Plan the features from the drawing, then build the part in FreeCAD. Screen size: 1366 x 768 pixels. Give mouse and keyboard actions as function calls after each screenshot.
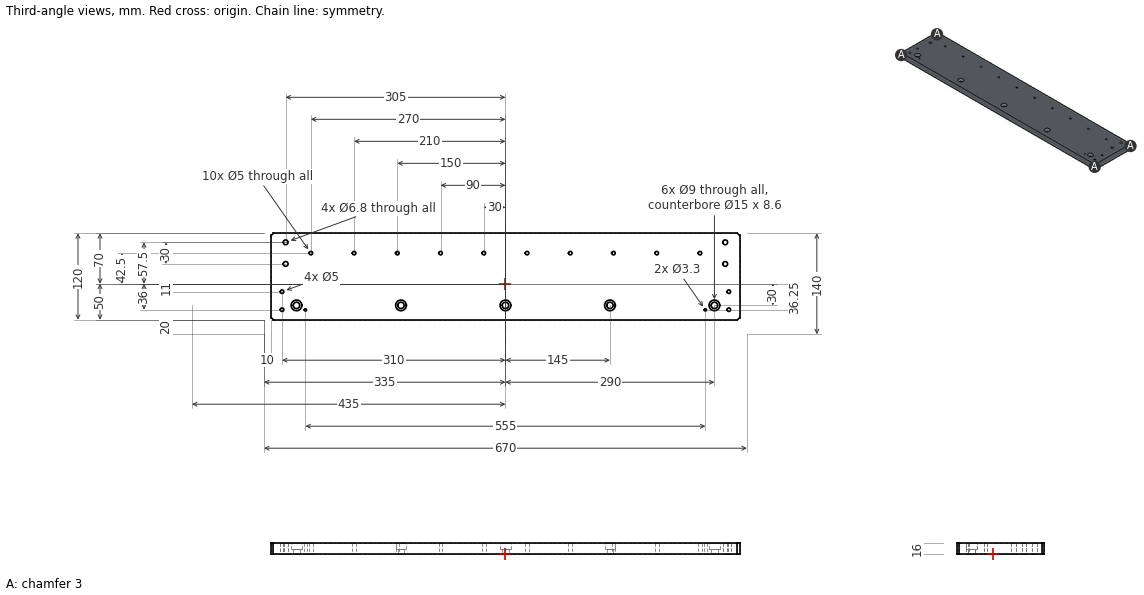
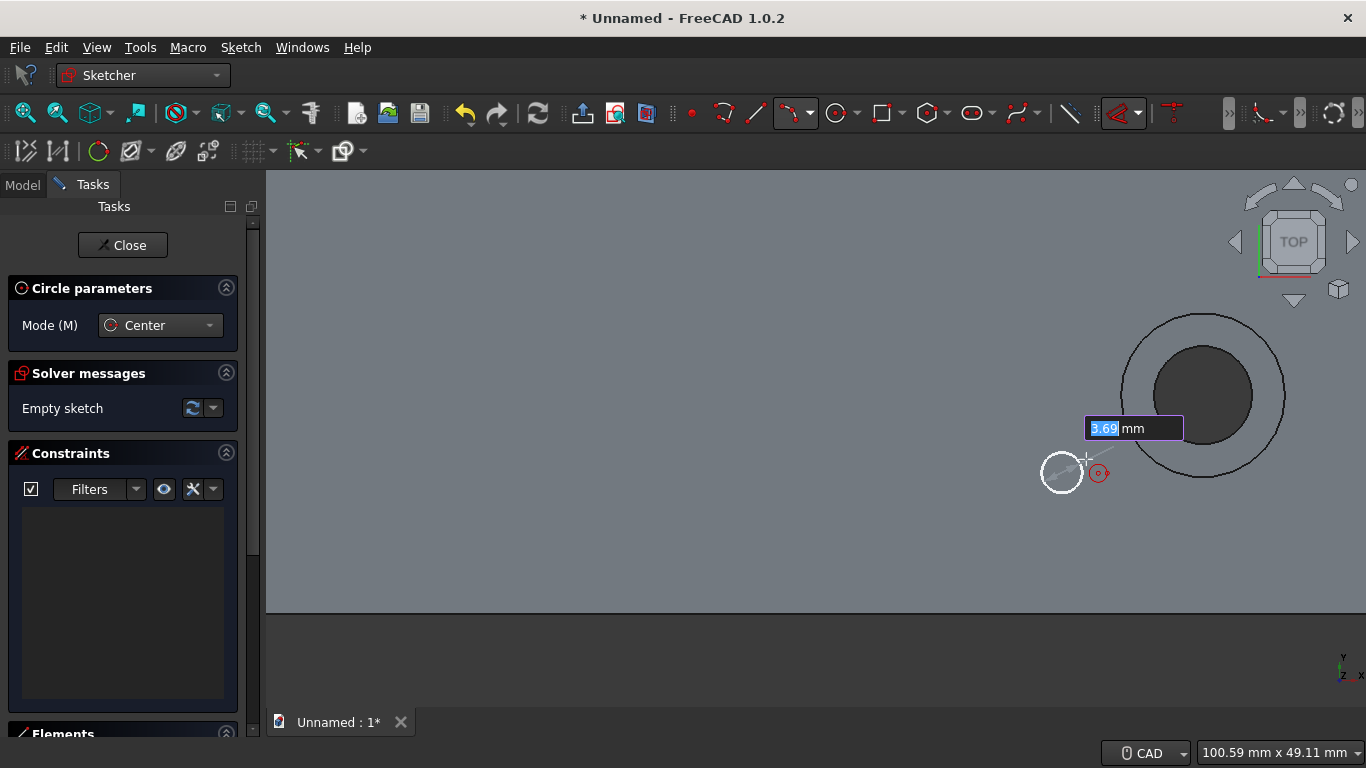
click(1079, 451)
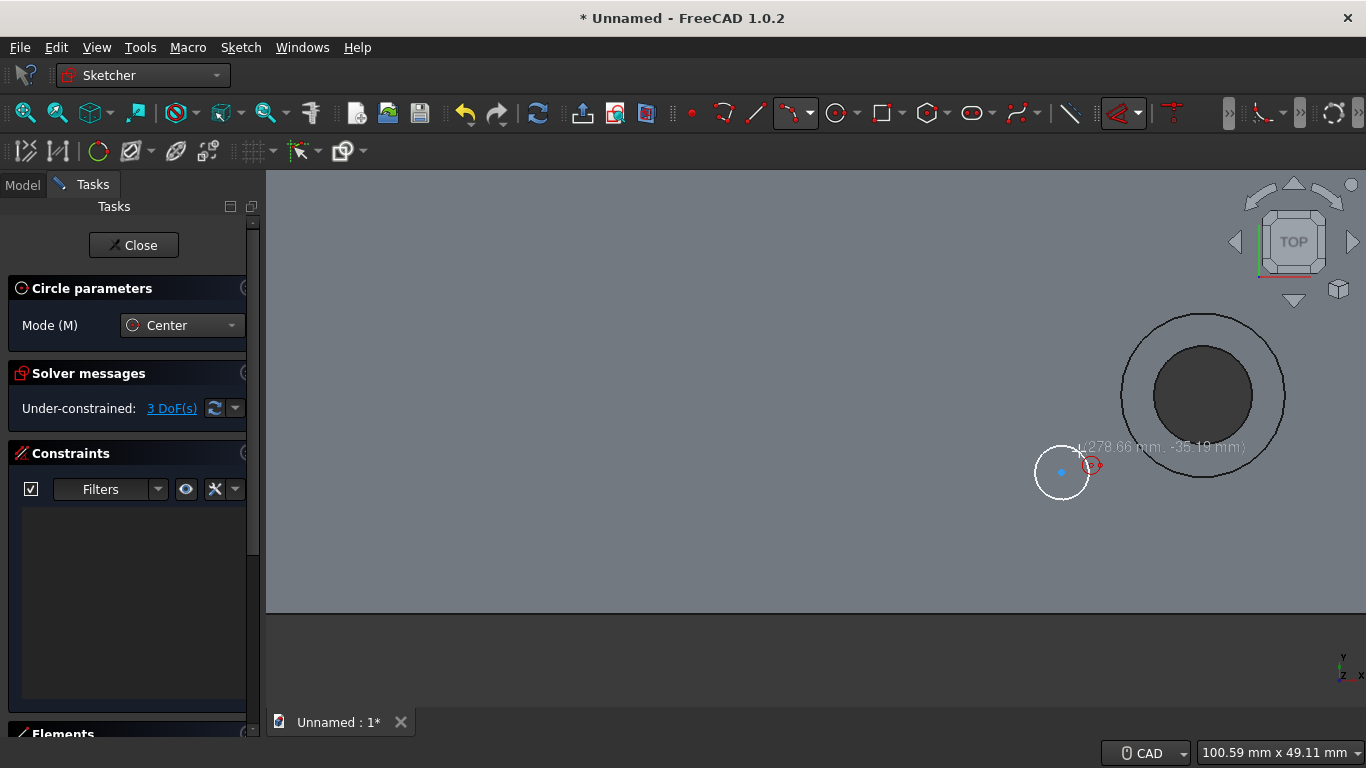
scroll(1086, 459, down, 11)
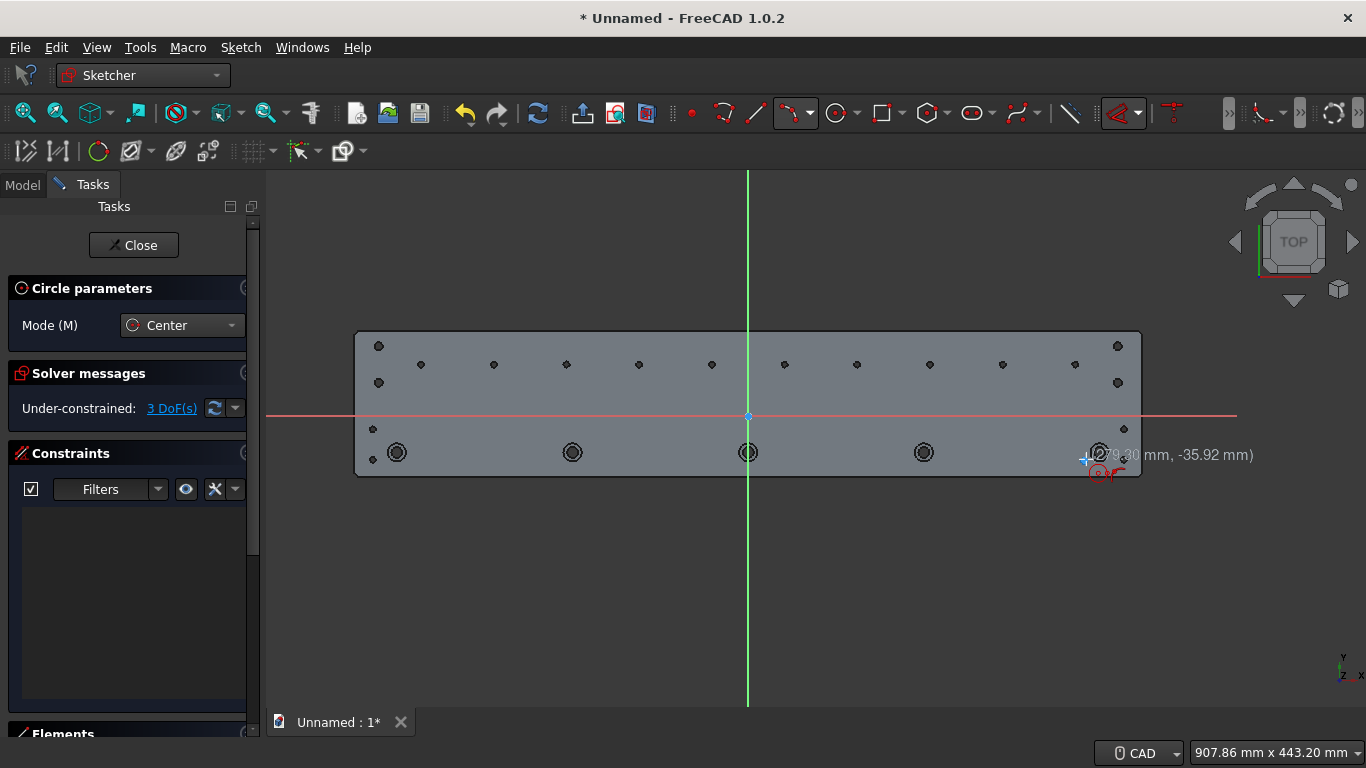
scroll(412, 460, up, 13)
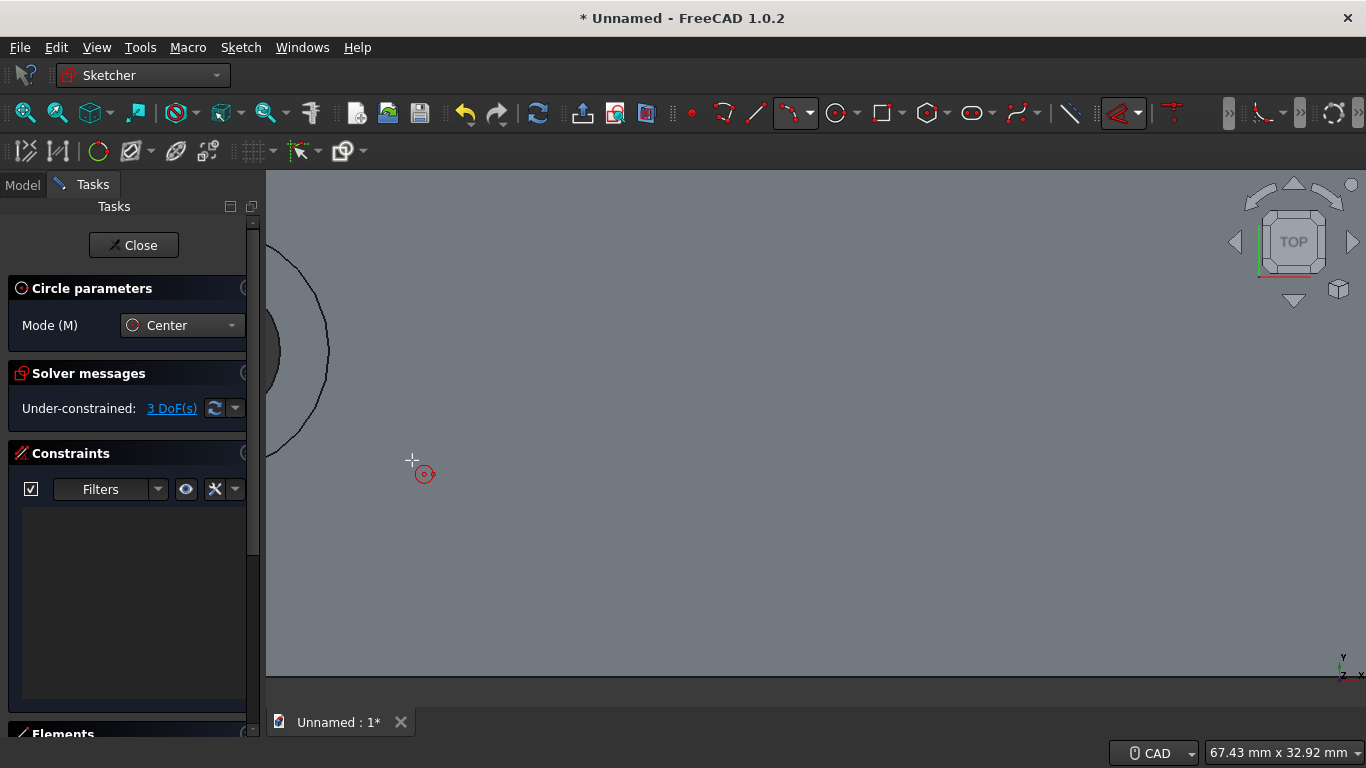
scroll(411, 460, down, 13)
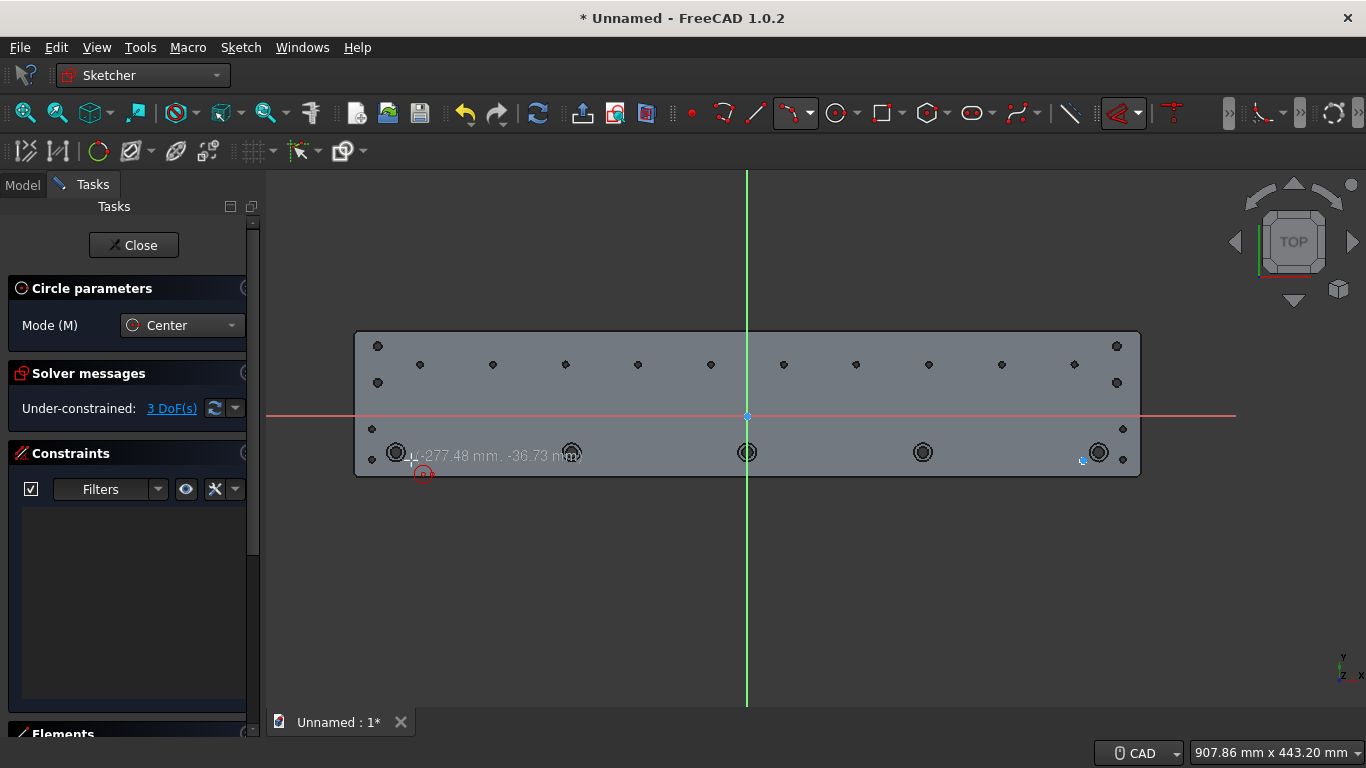
click(411, 460)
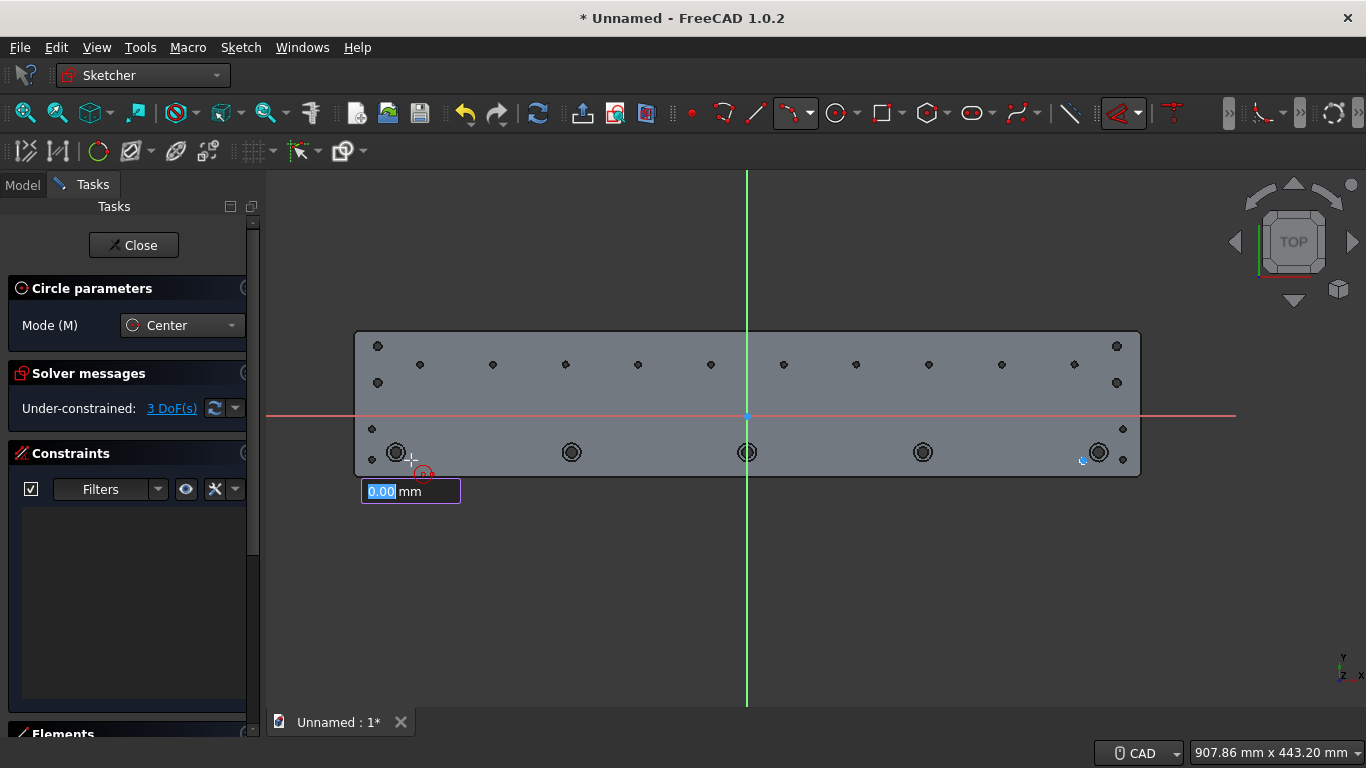
scroll(413, 459, up, 11)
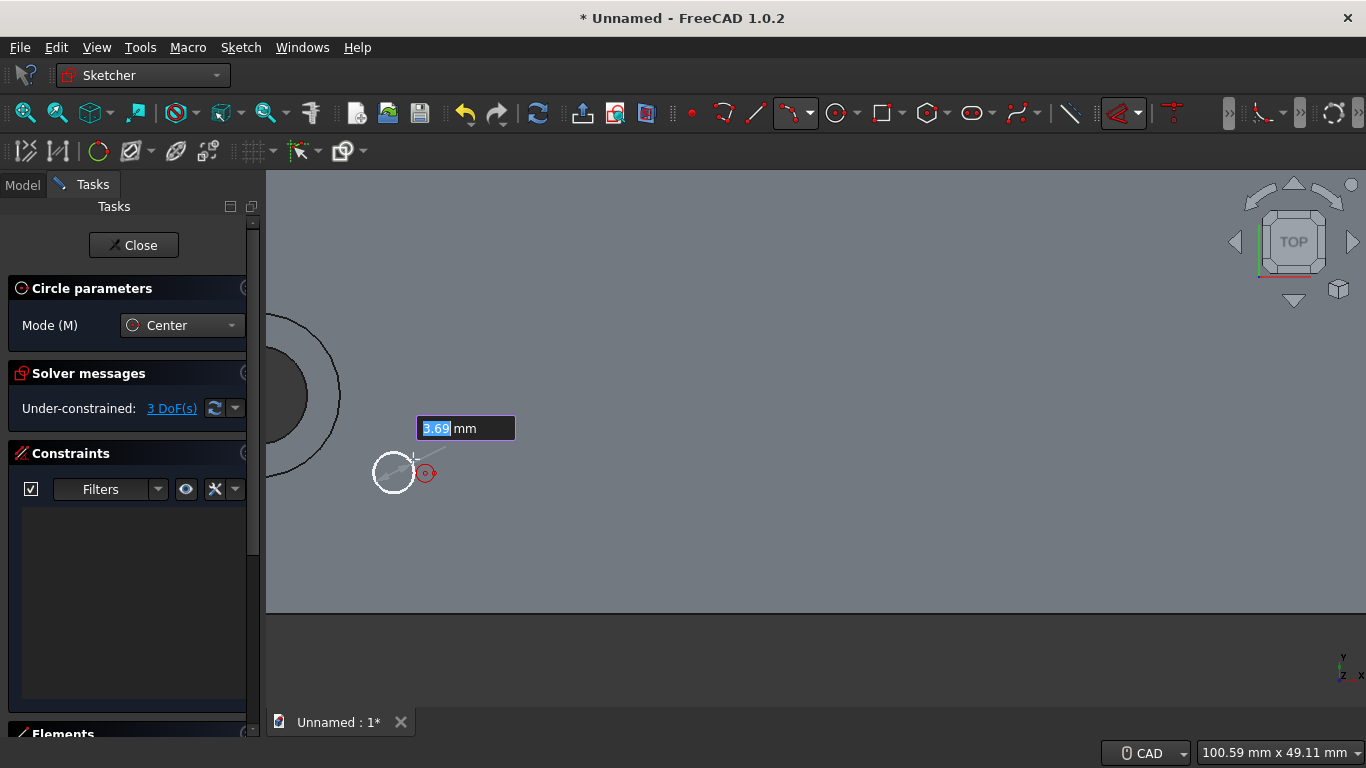
click(408, 451)
key(Escape)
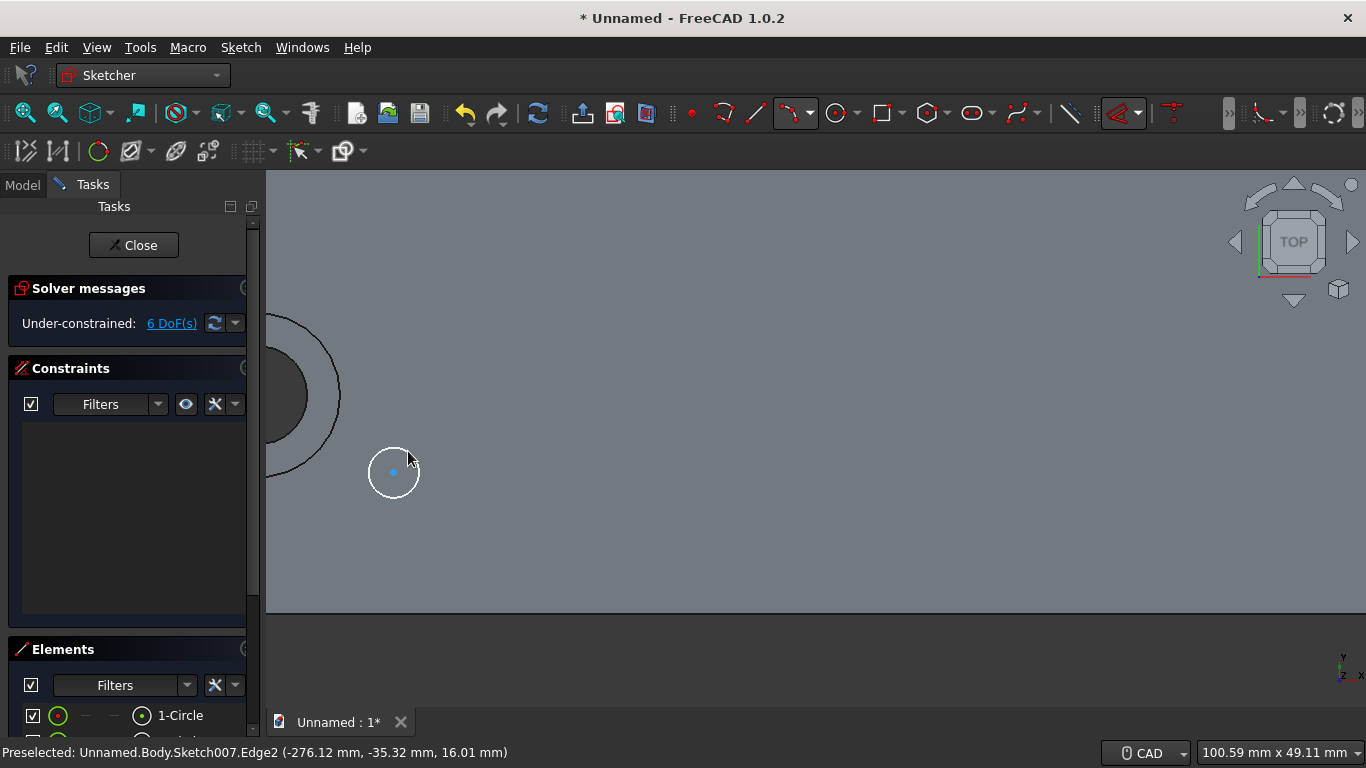
scroll(413, 459, down, 11)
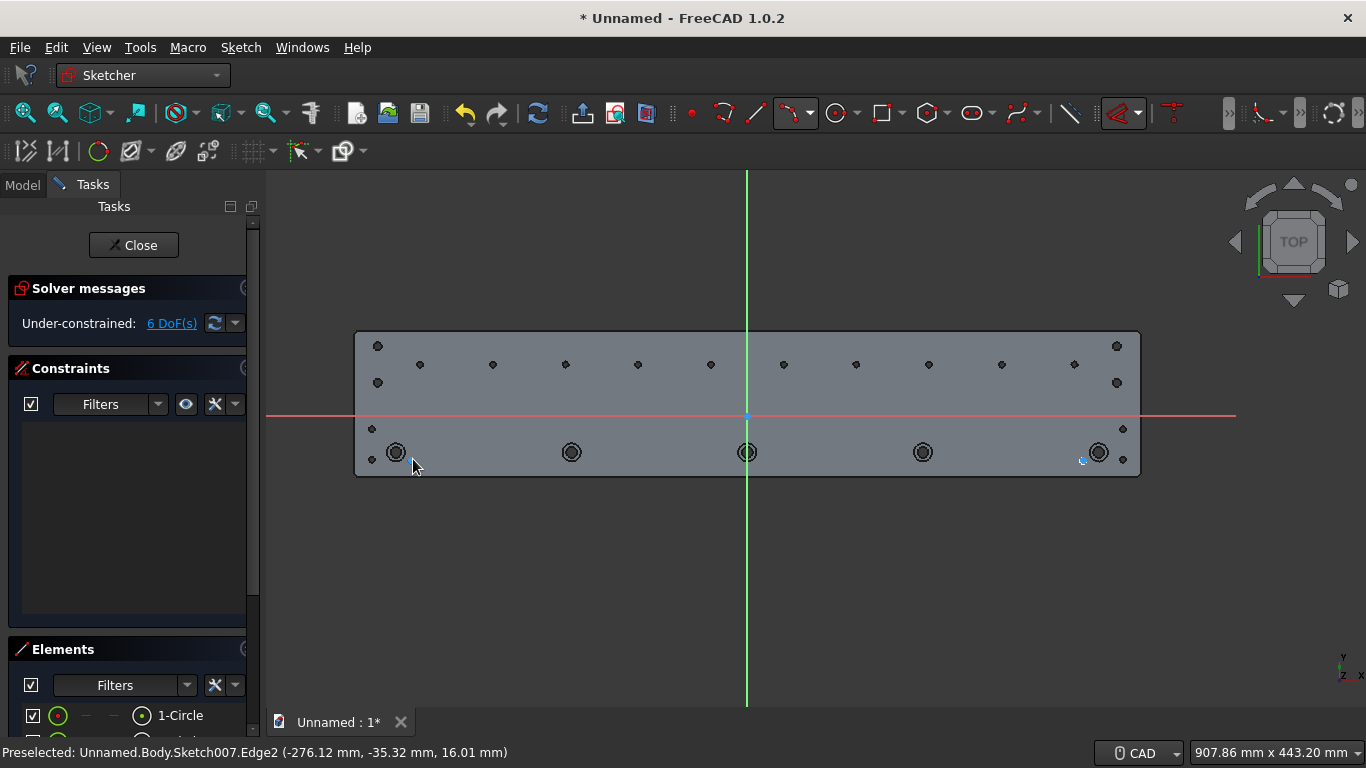
scroll(1085, 459, up, 8)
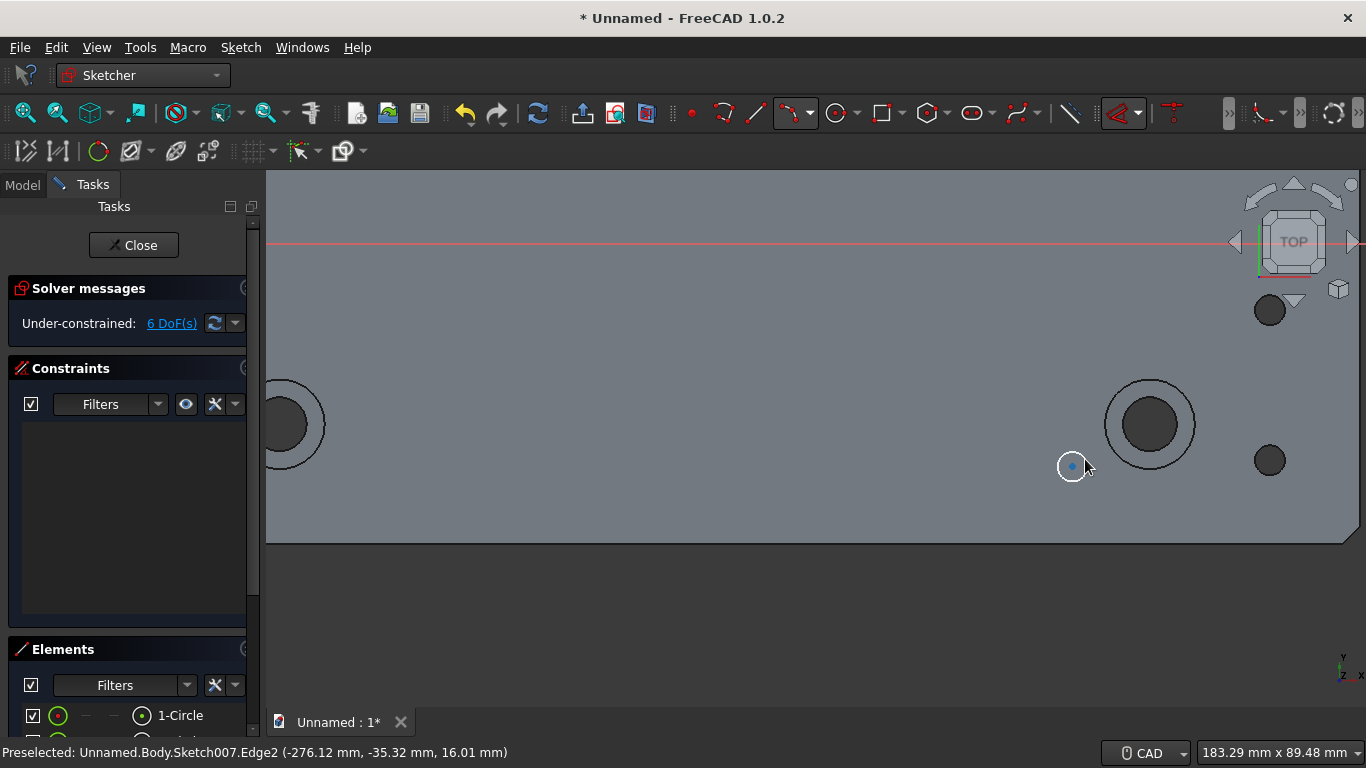
click(1083, 456)